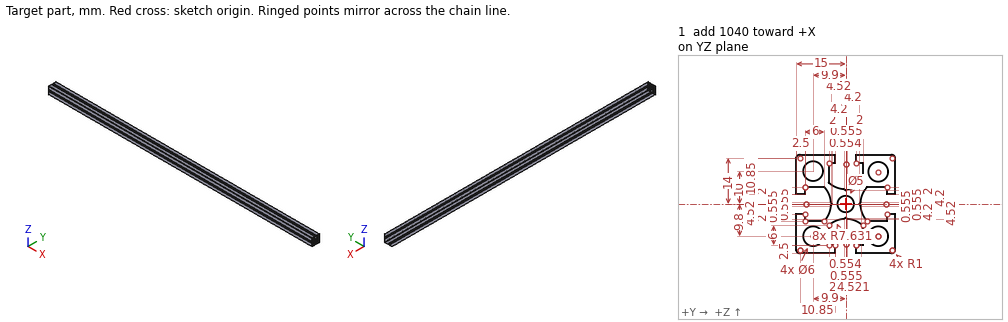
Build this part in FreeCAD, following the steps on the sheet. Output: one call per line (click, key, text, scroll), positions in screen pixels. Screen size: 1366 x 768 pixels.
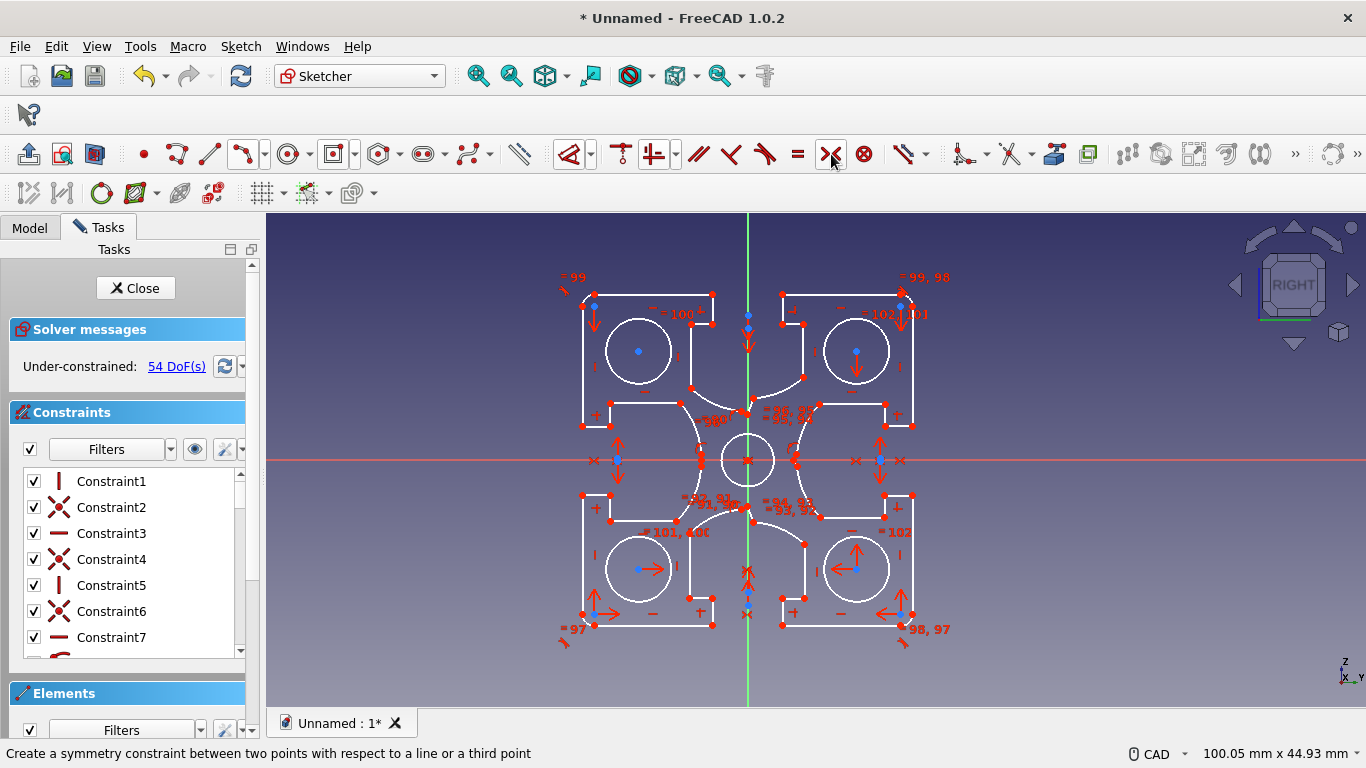
click(610, 403)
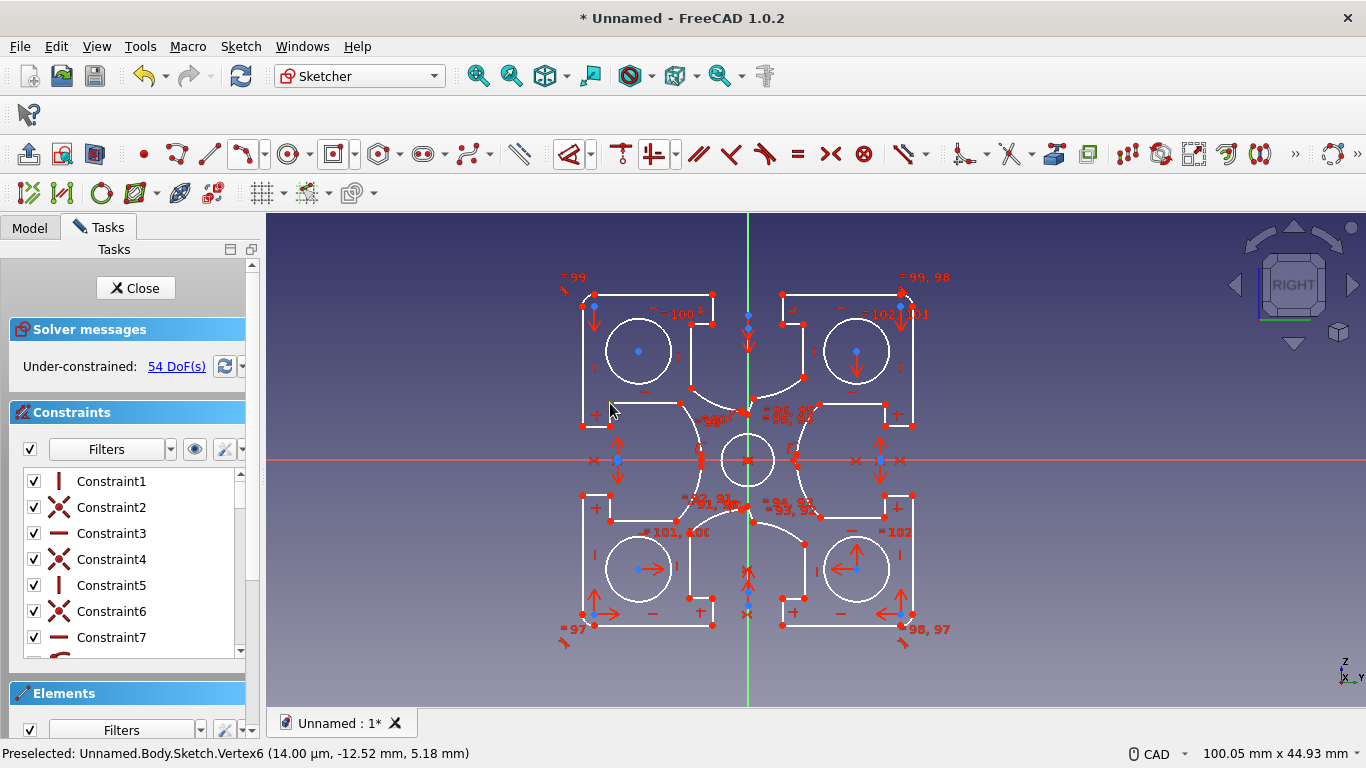
click(610, 521)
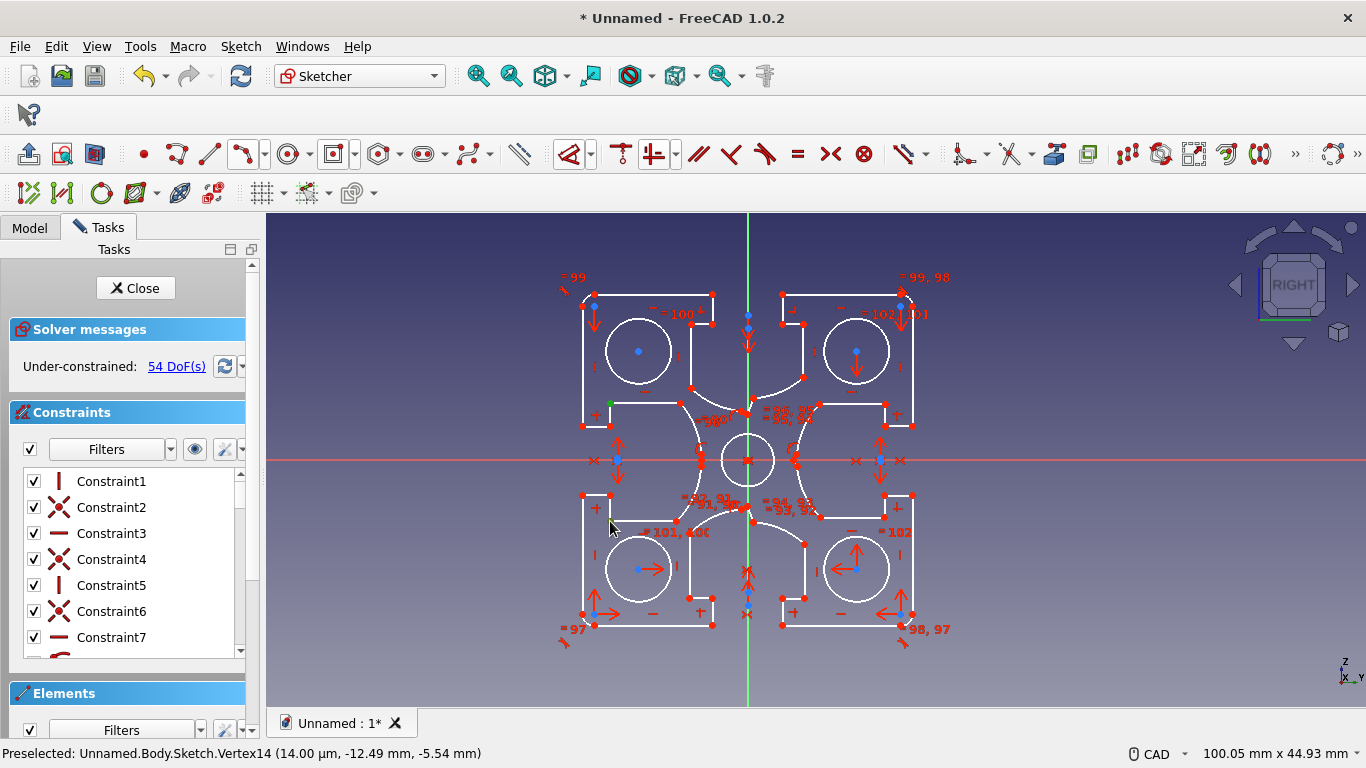
click(359, 460)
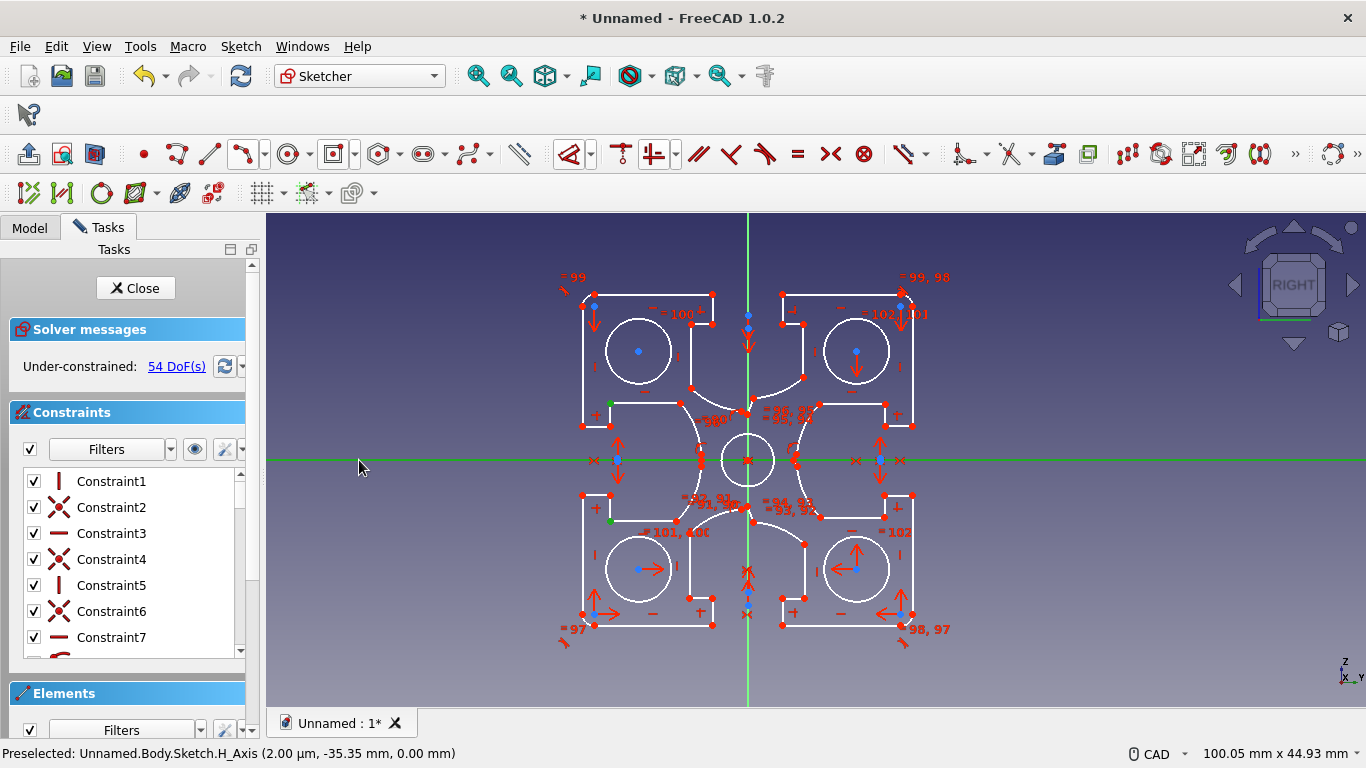
click(831, 154)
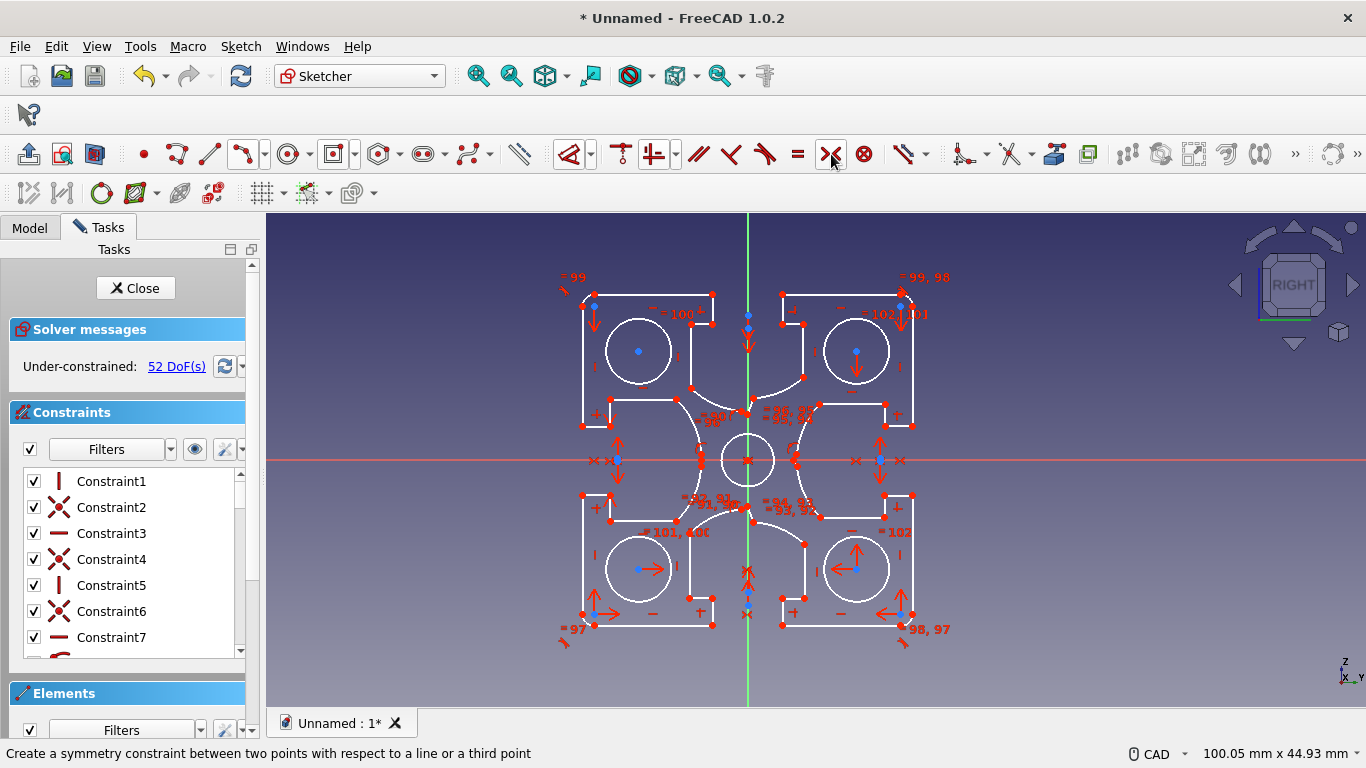
click(690, 534)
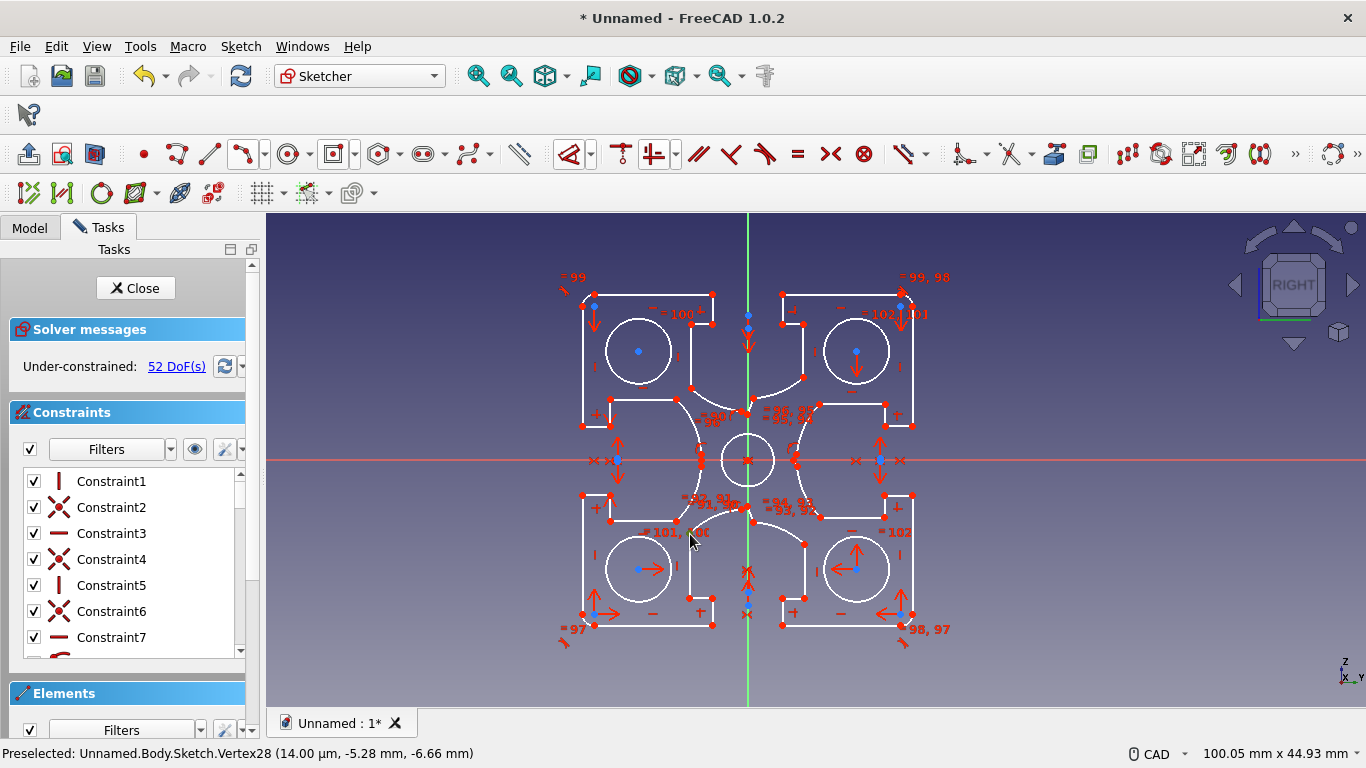
click(805, 544)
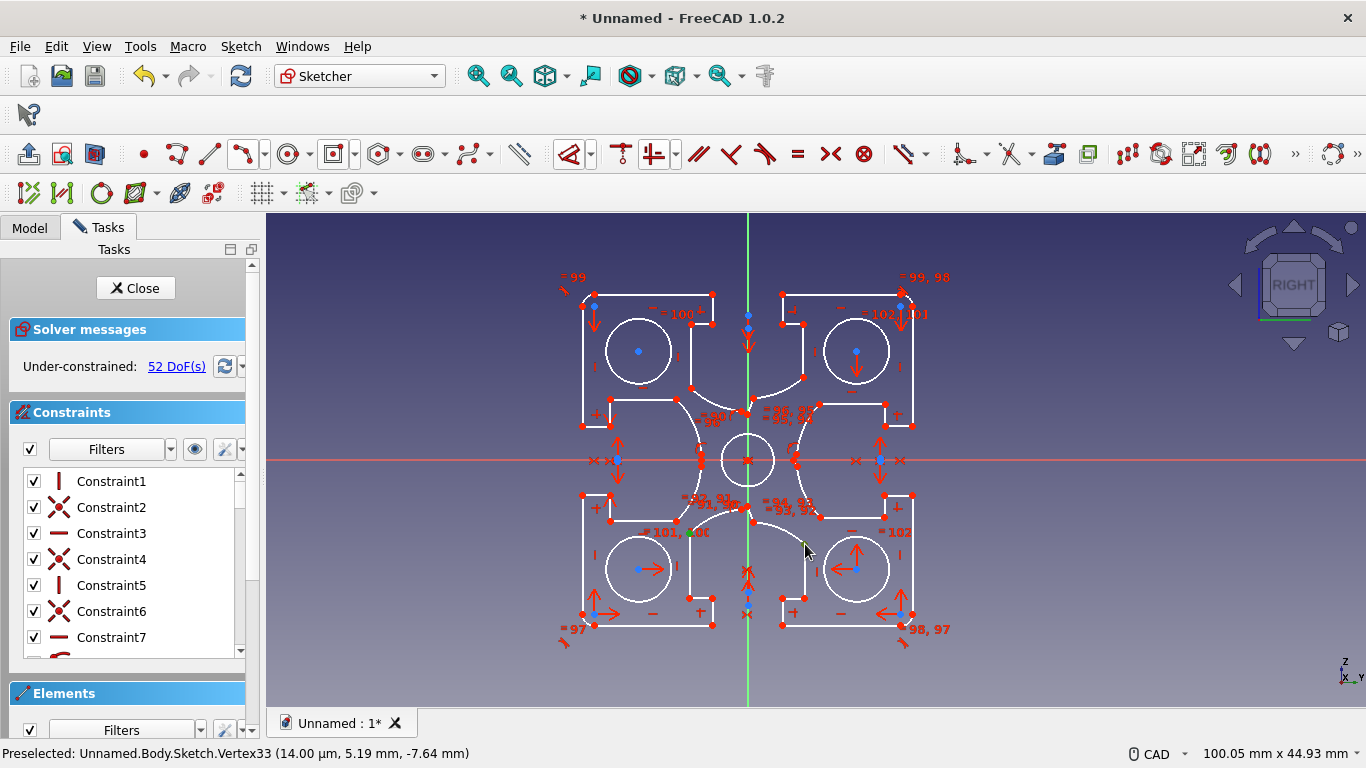
click(748, 648)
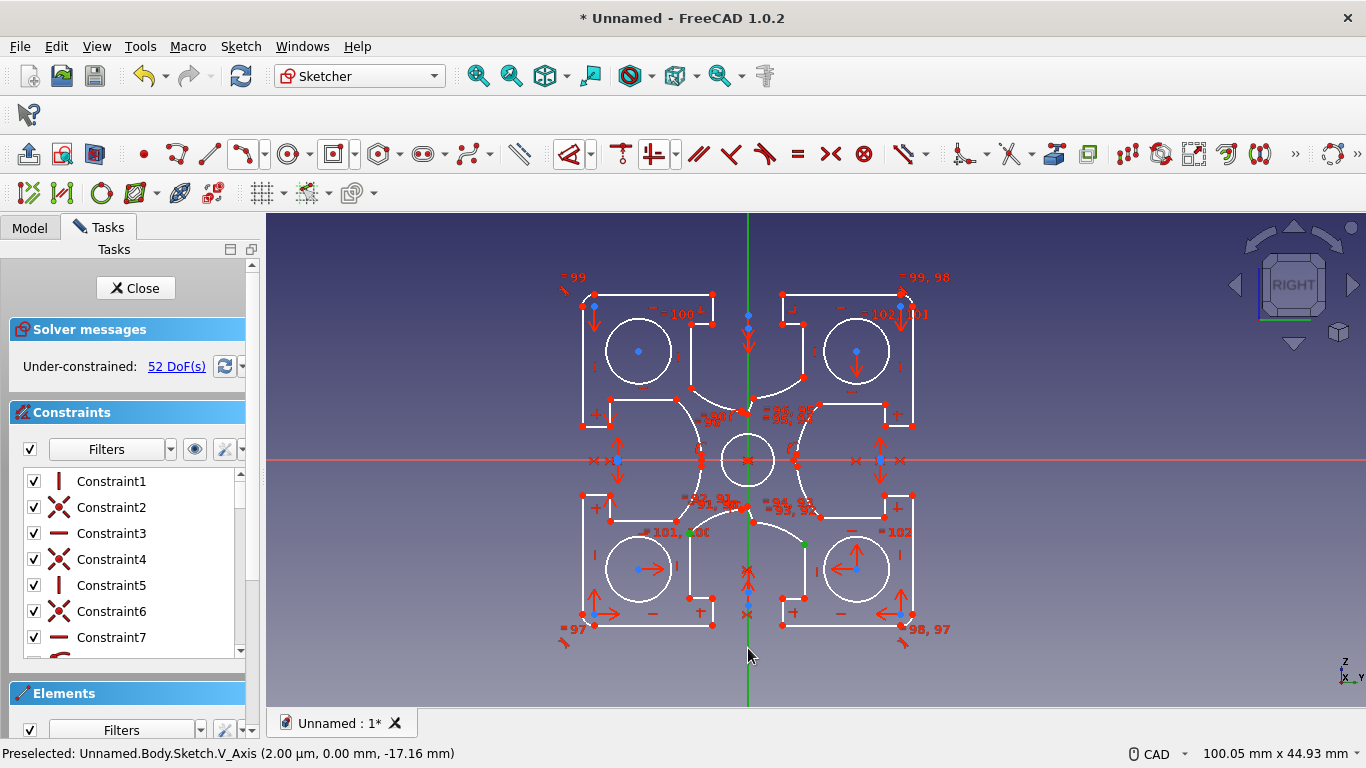
click(831, 154)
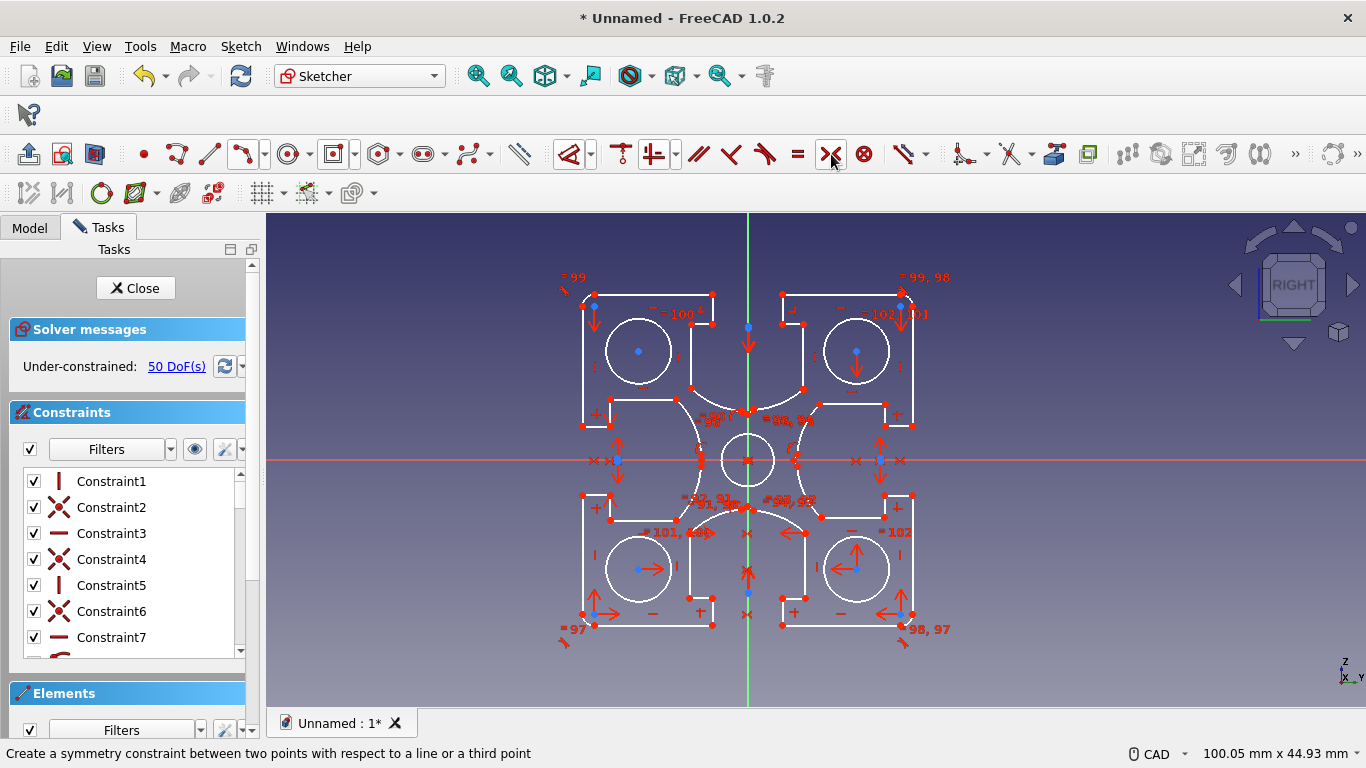
click(713, 598)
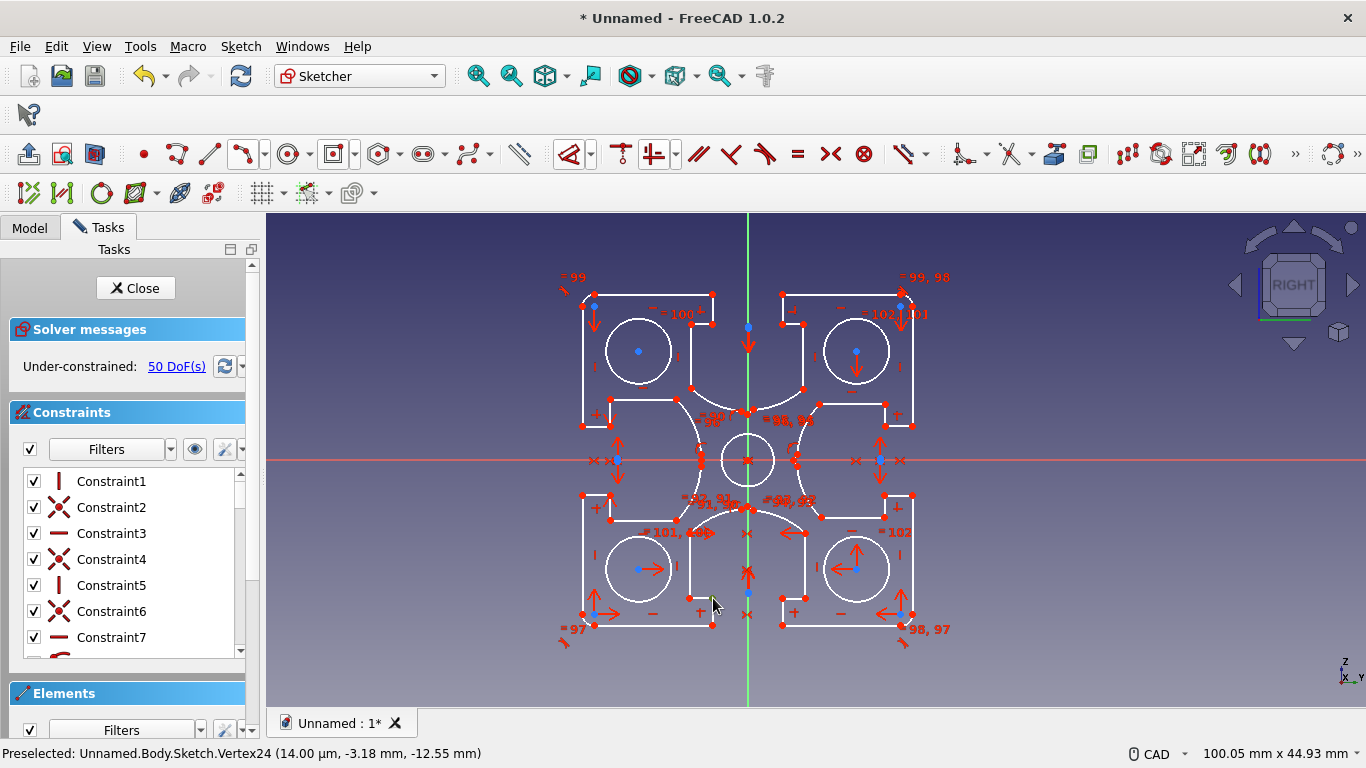
click(783, 599)